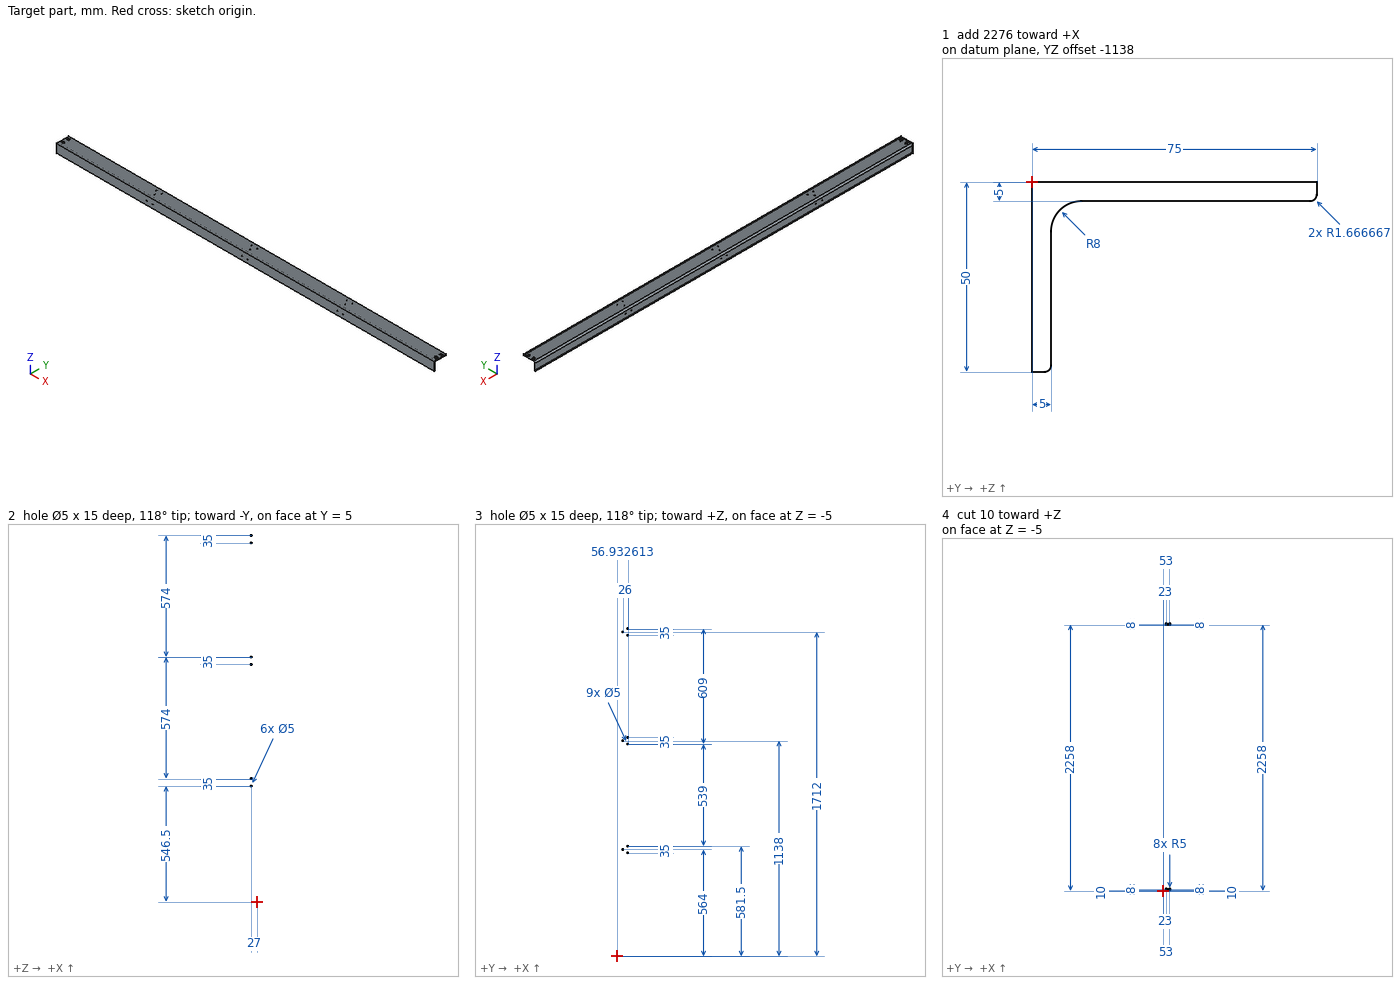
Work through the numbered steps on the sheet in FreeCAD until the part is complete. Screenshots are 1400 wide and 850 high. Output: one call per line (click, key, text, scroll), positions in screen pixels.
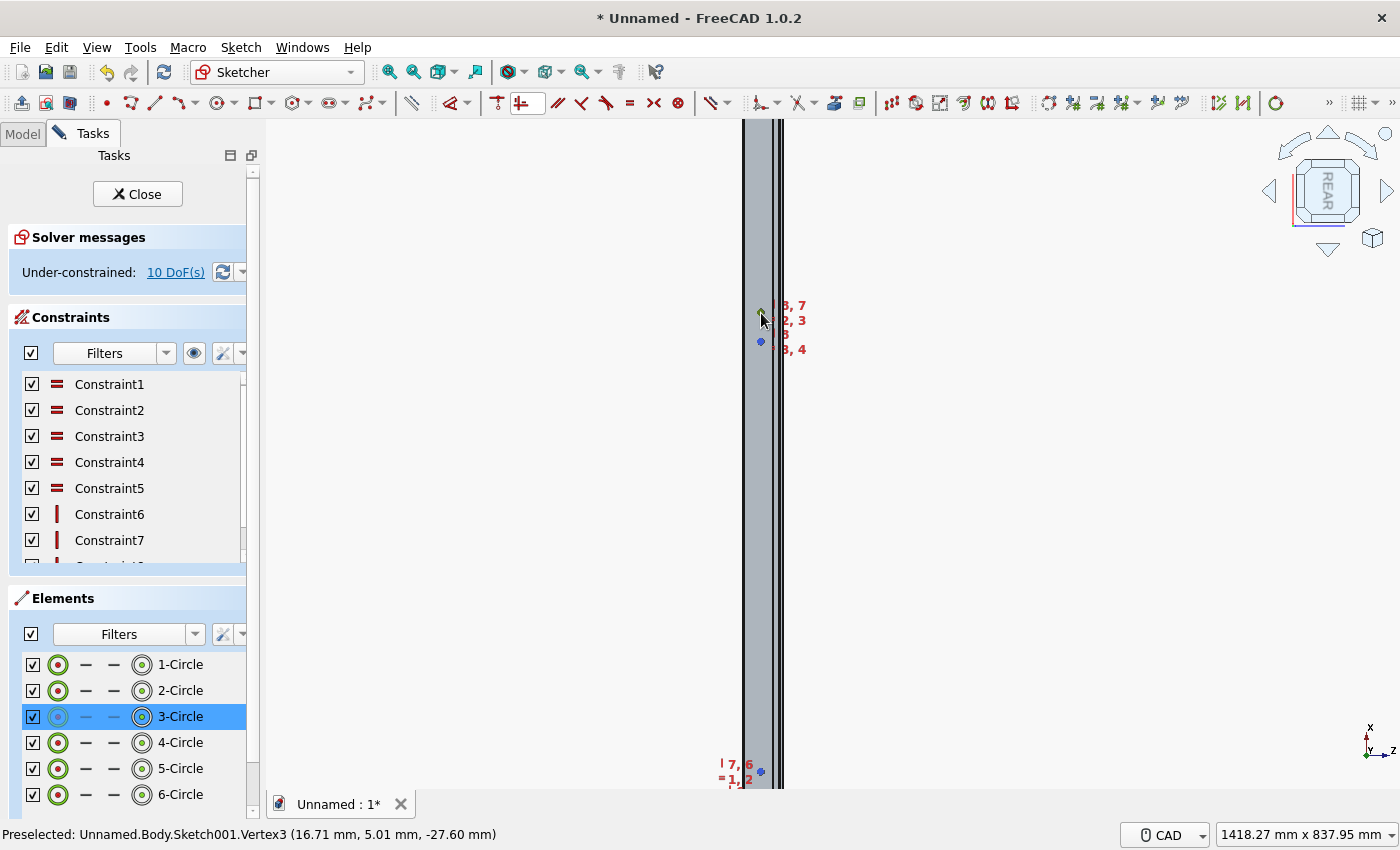
scroll(762, 415, down, 6)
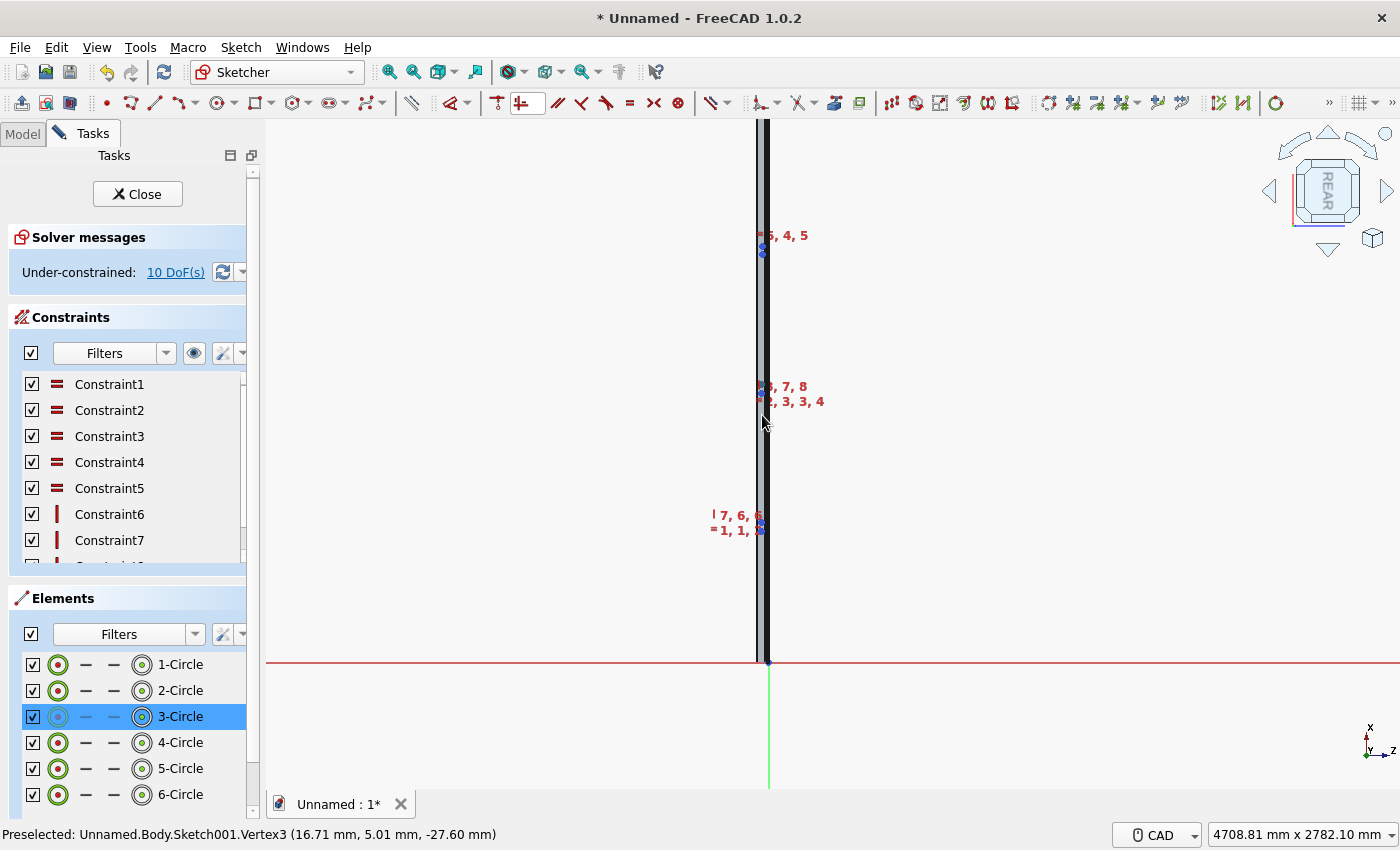
scroll(762, 246, up, 2)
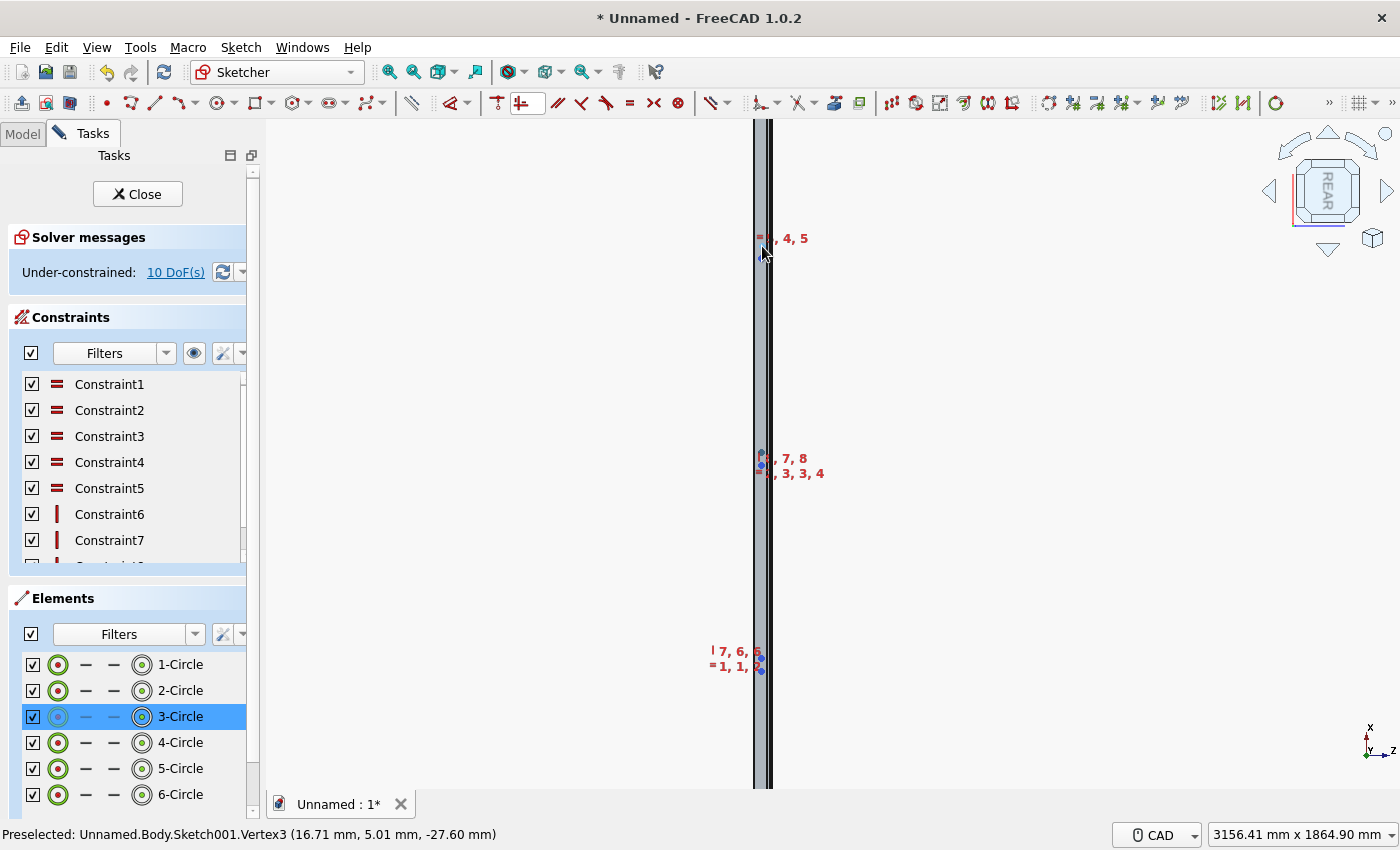
click(762, 246)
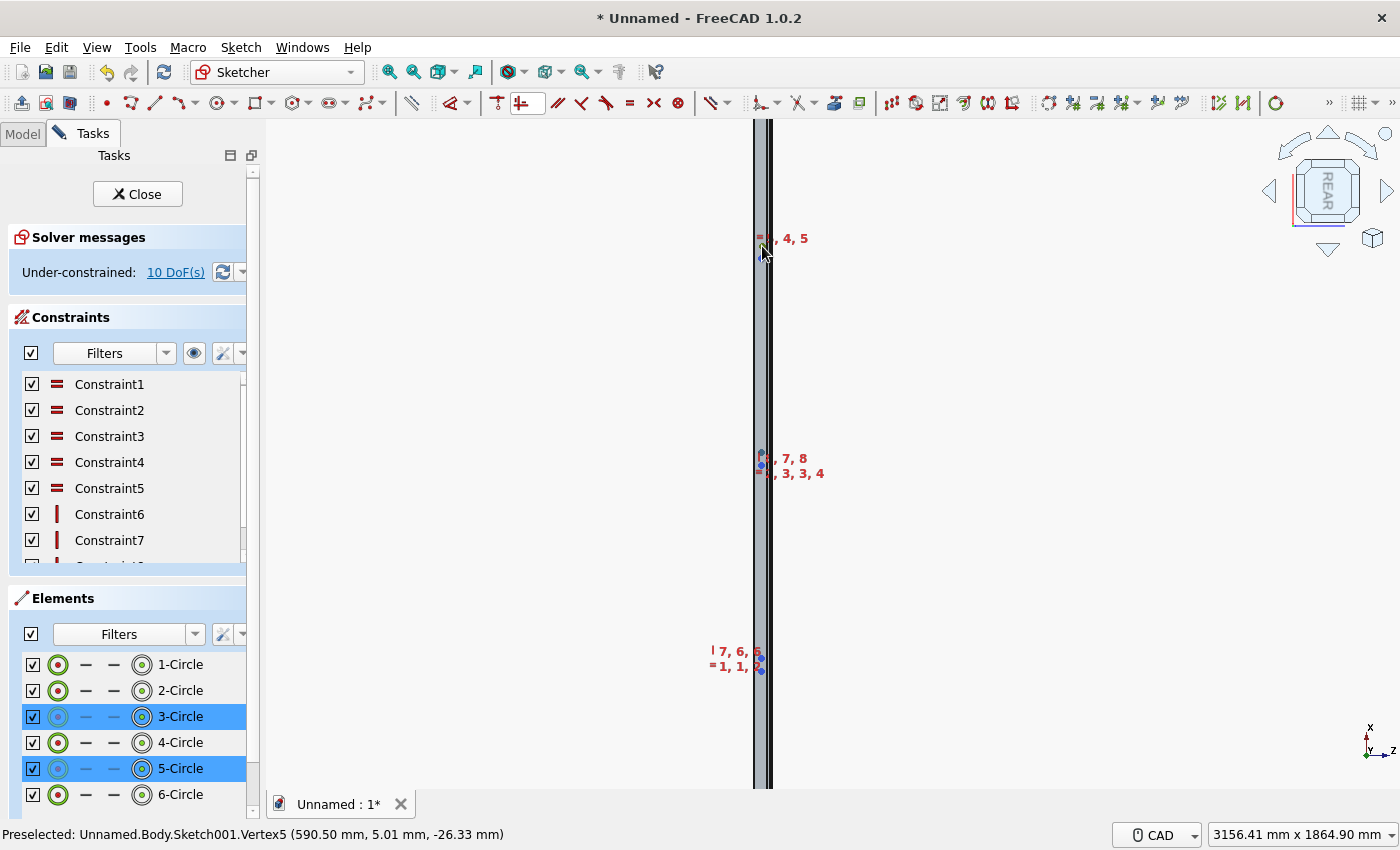
click(540, 104)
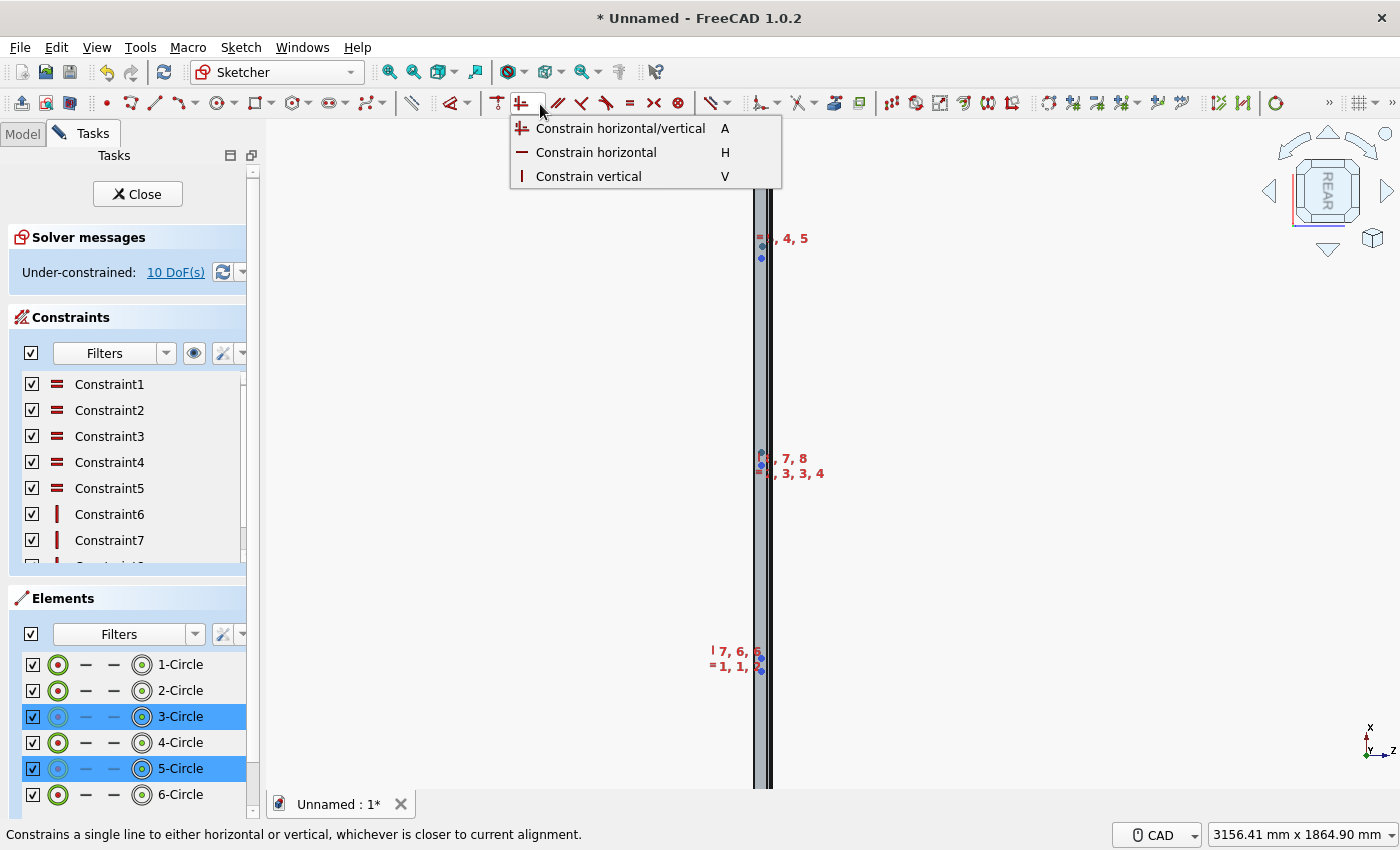
click(646, 176)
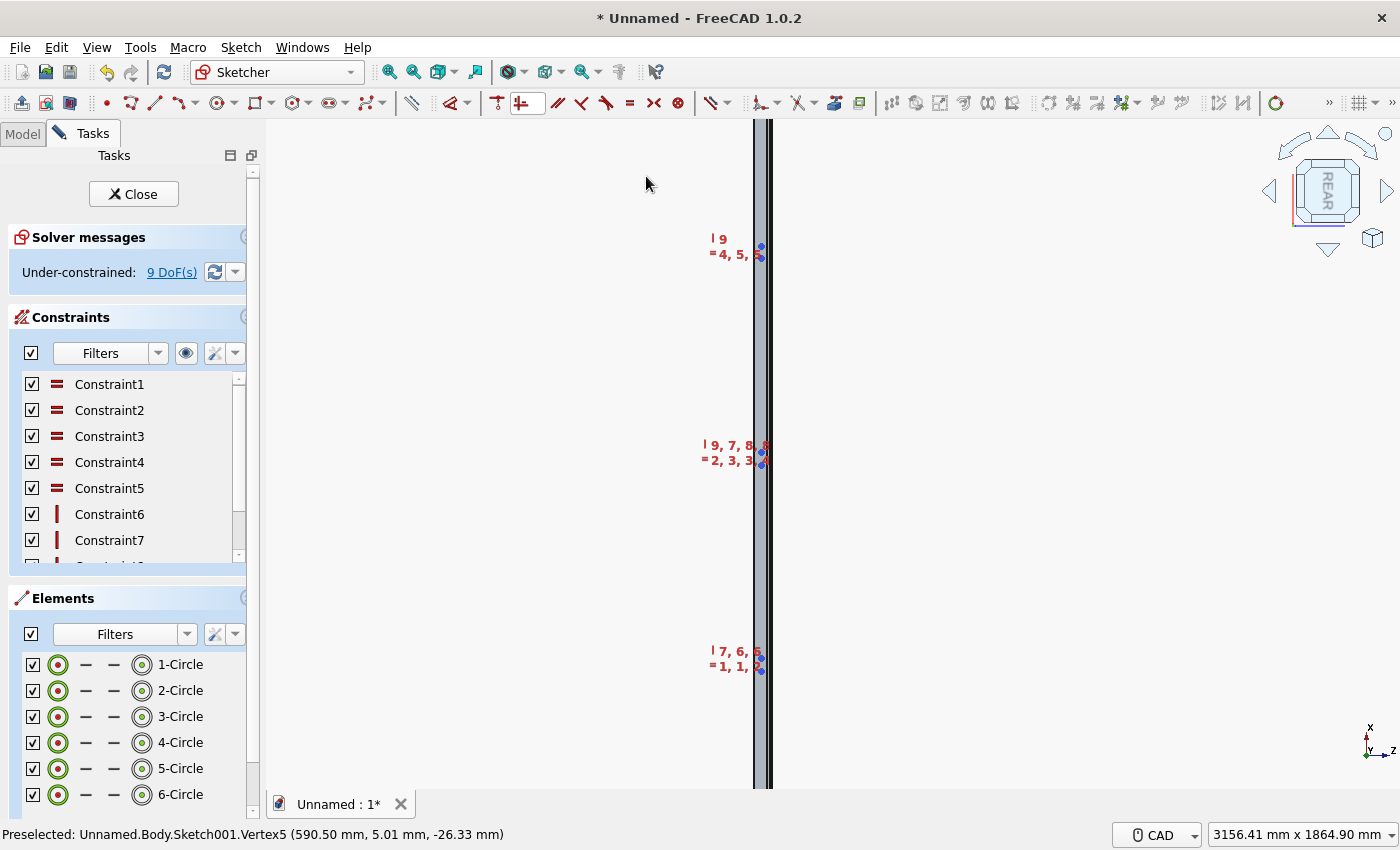
click(762, 246)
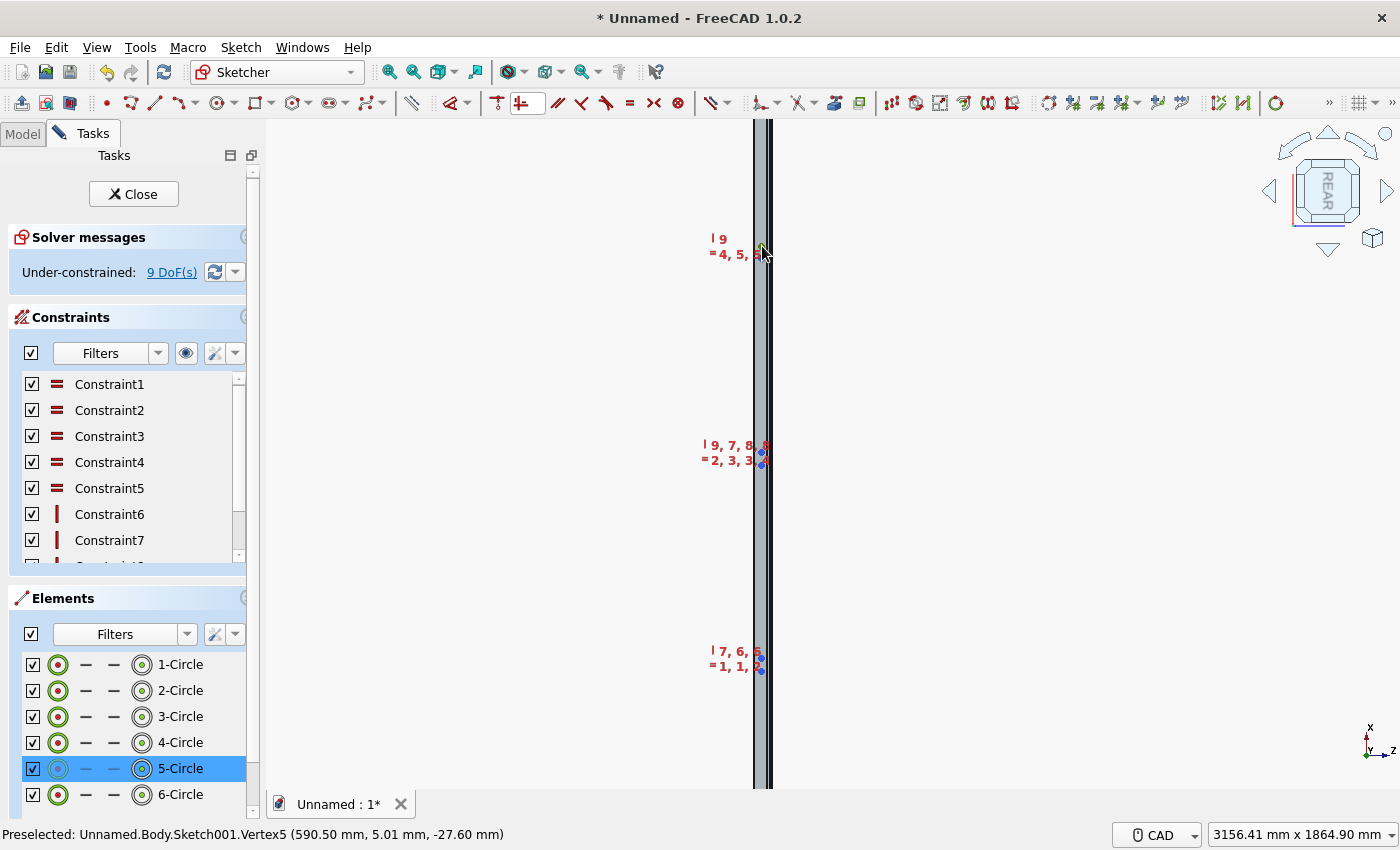
click(762, 259)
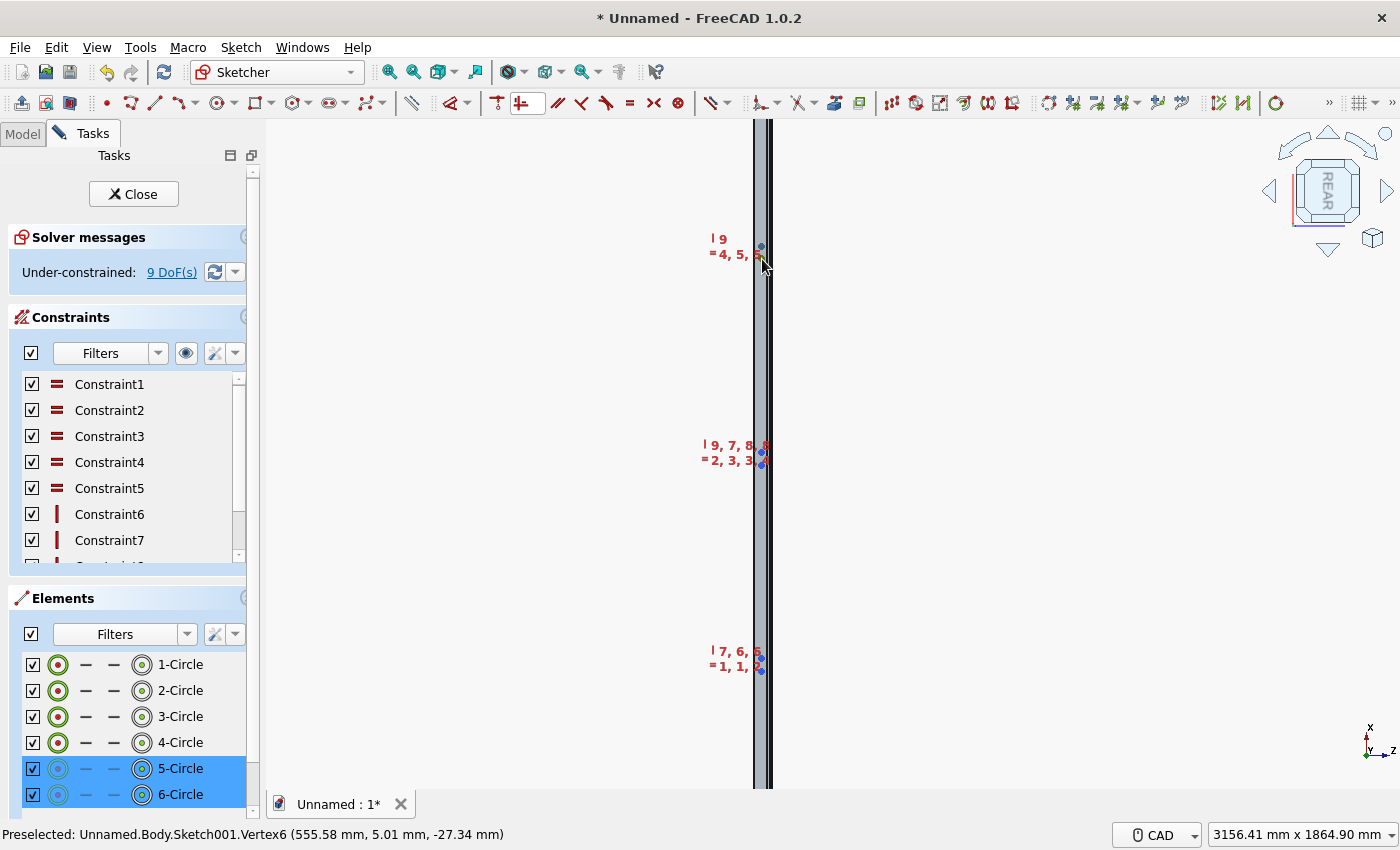
key(v)